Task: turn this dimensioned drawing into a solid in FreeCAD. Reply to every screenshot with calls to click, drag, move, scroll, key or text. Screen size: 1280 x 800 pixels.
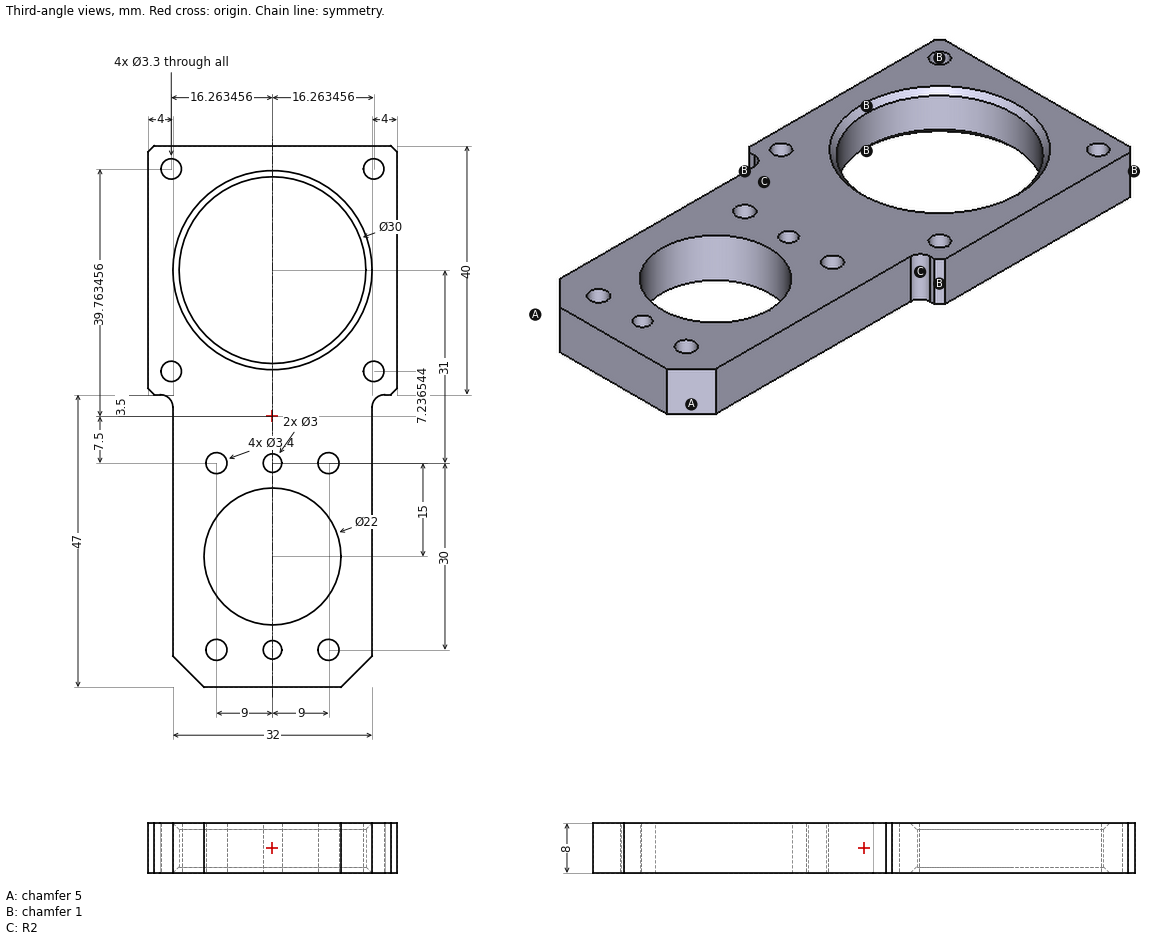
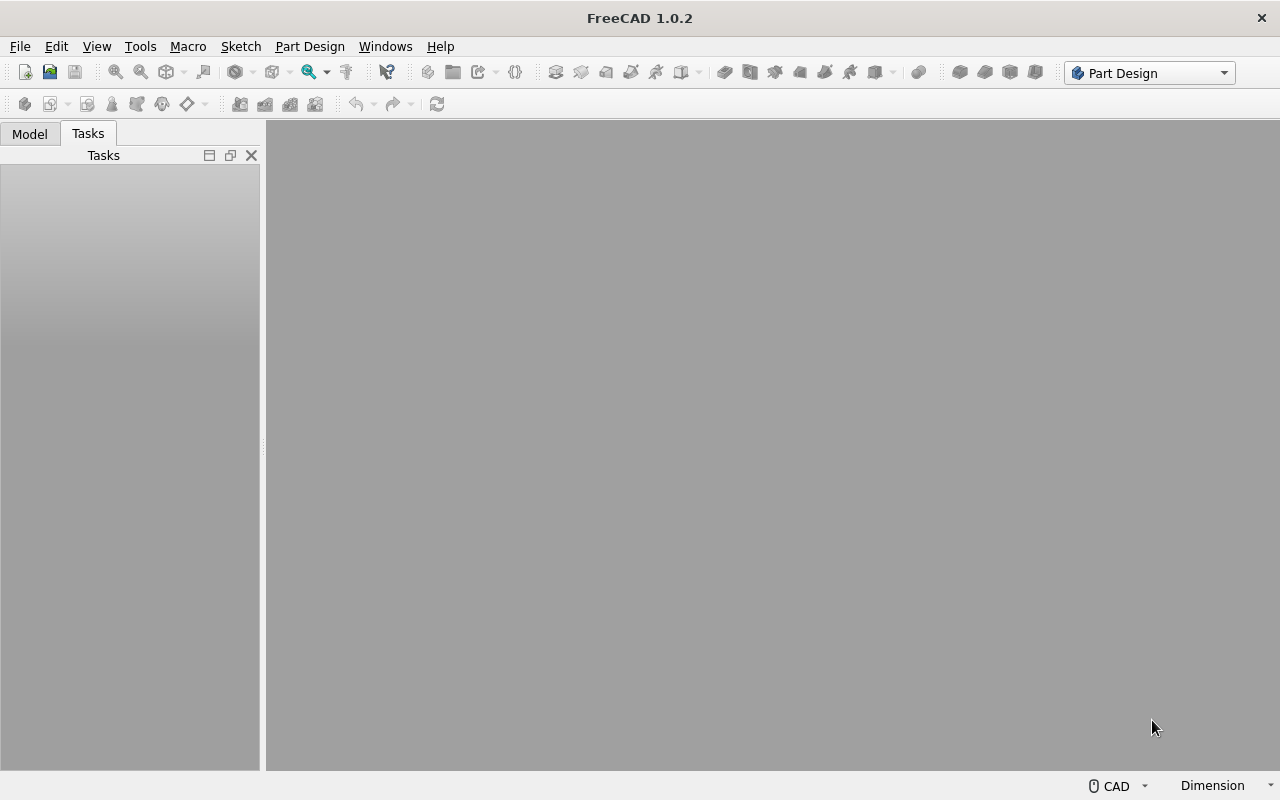
click(25, 72)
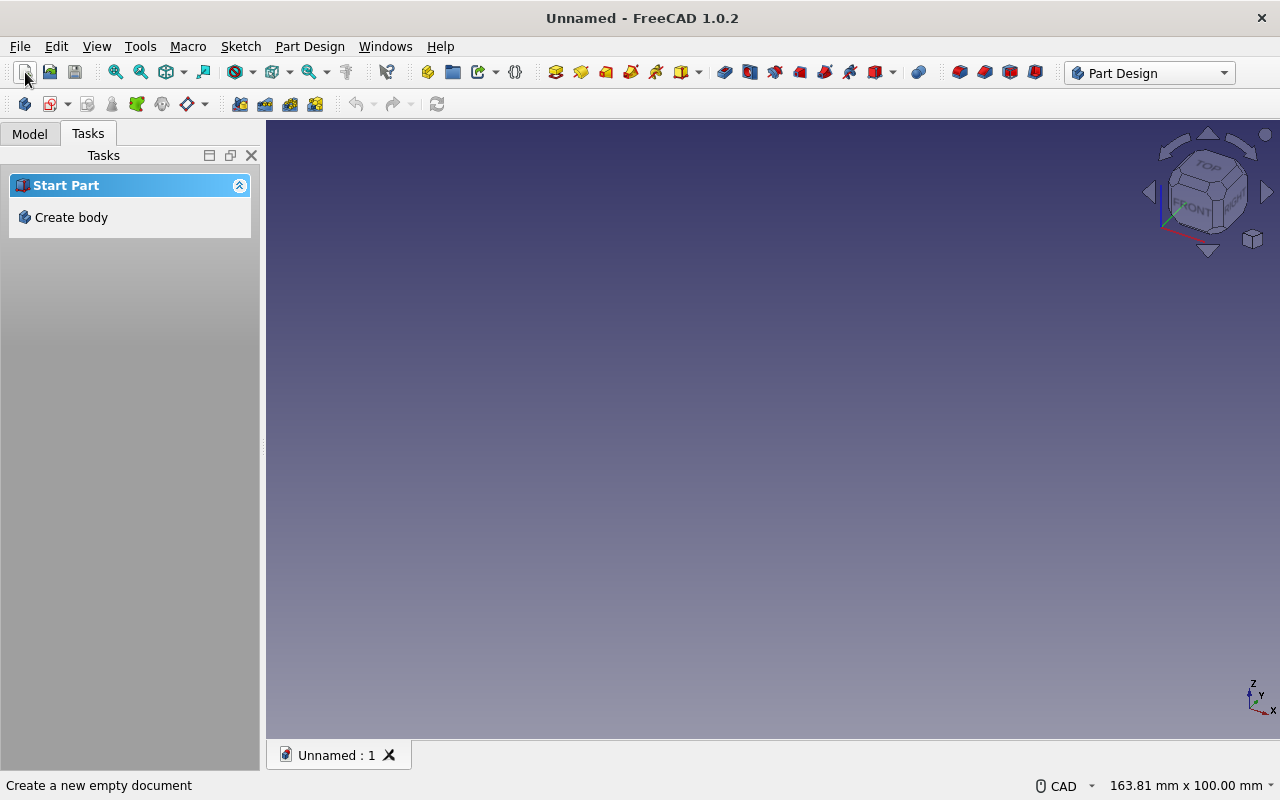
click(50, 104)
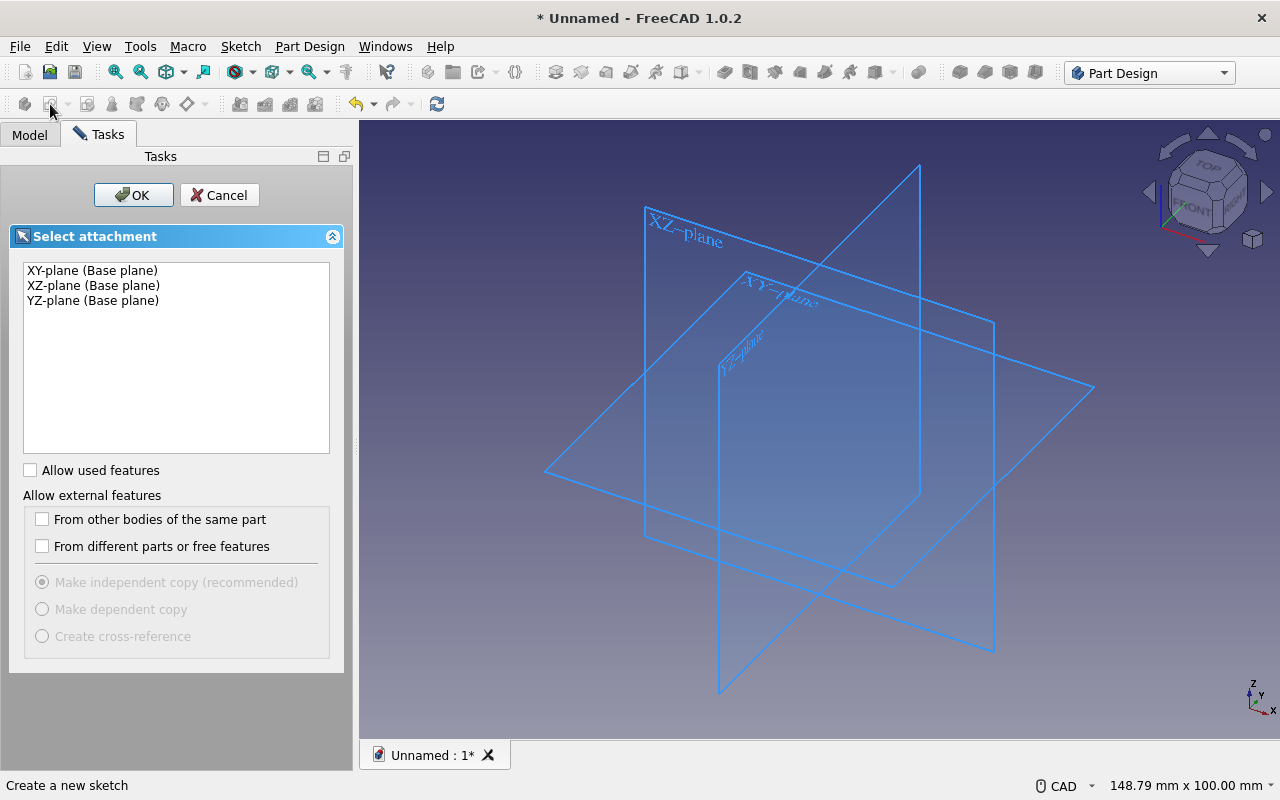
click(84, 270)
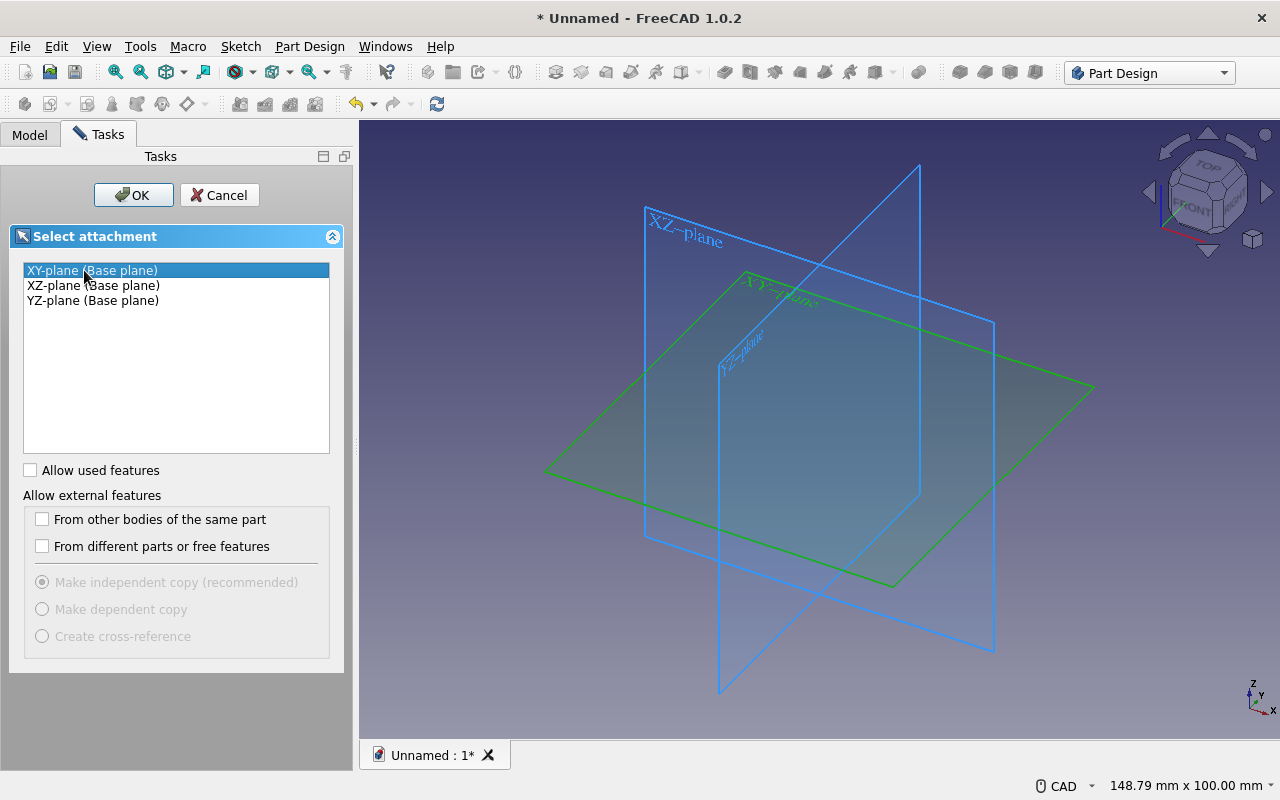
click(134, 195)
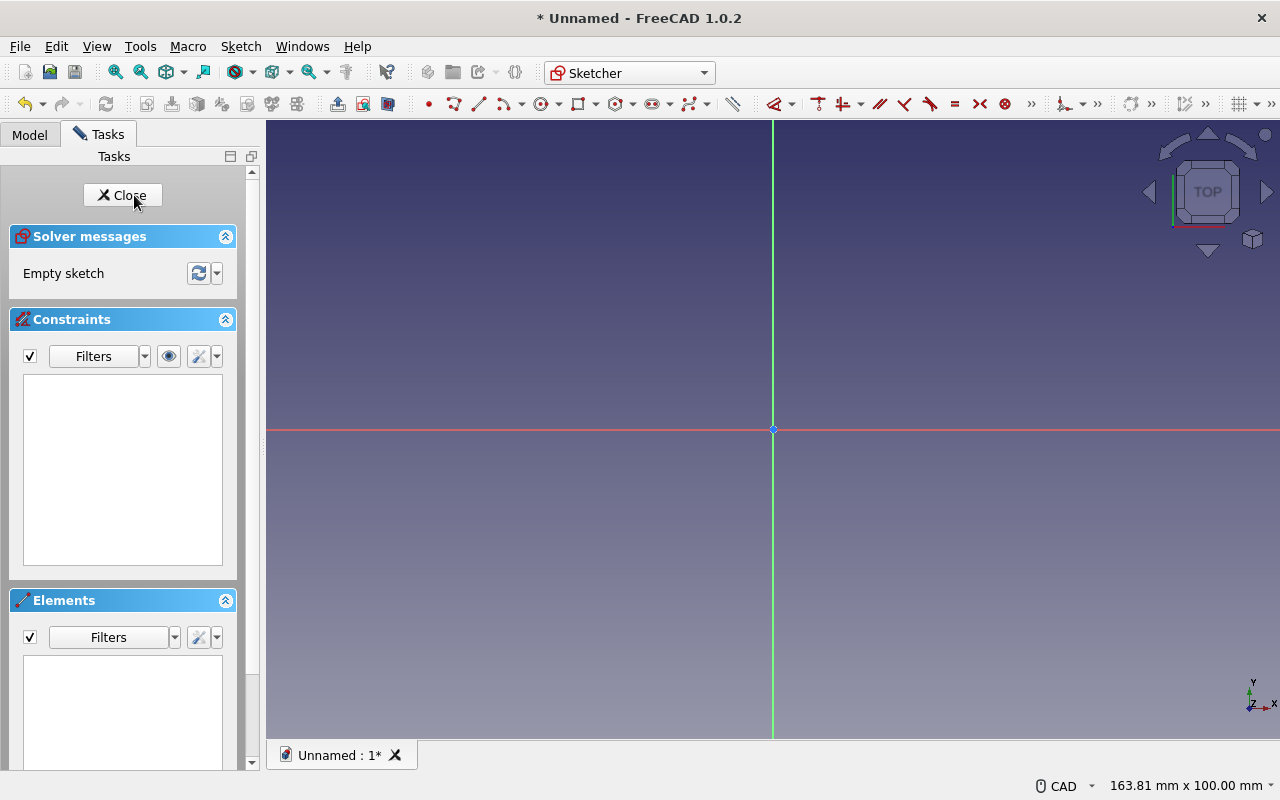
scroll(565, 429, down, 2)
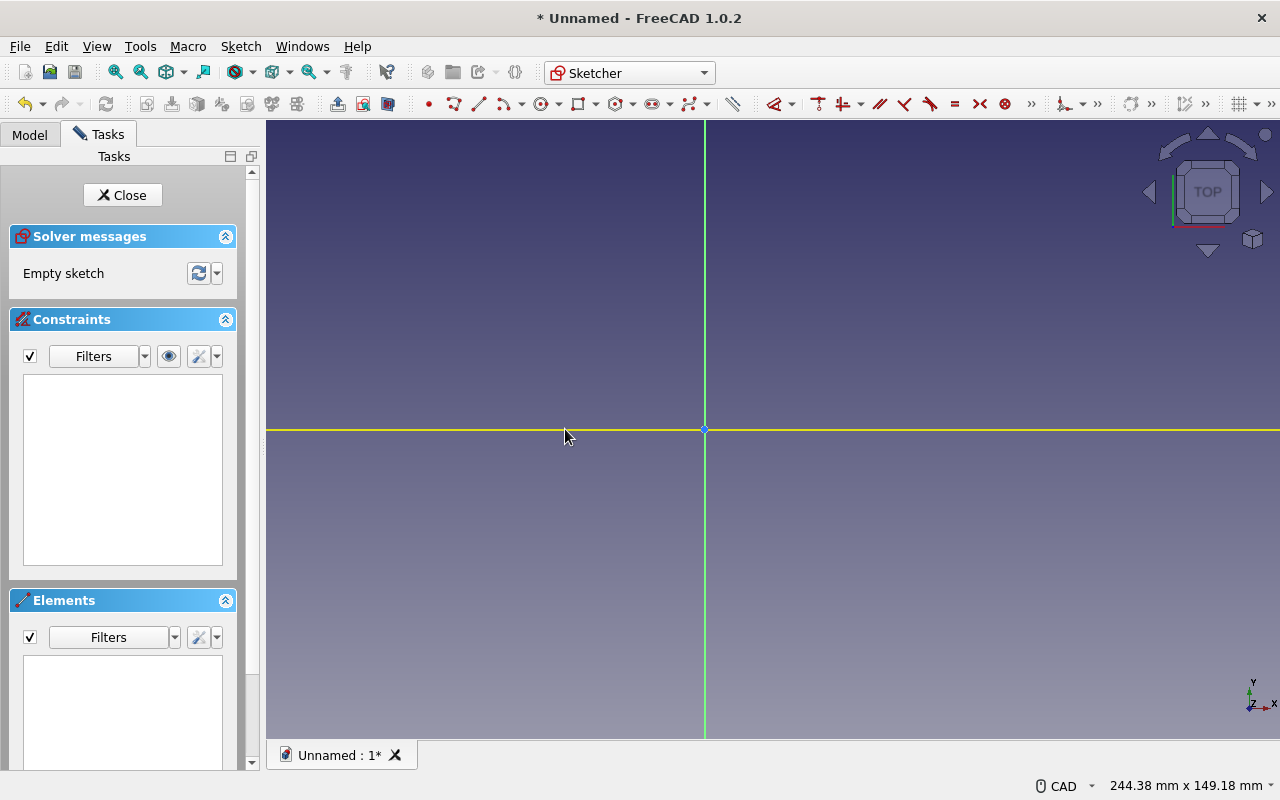
click(454, 104)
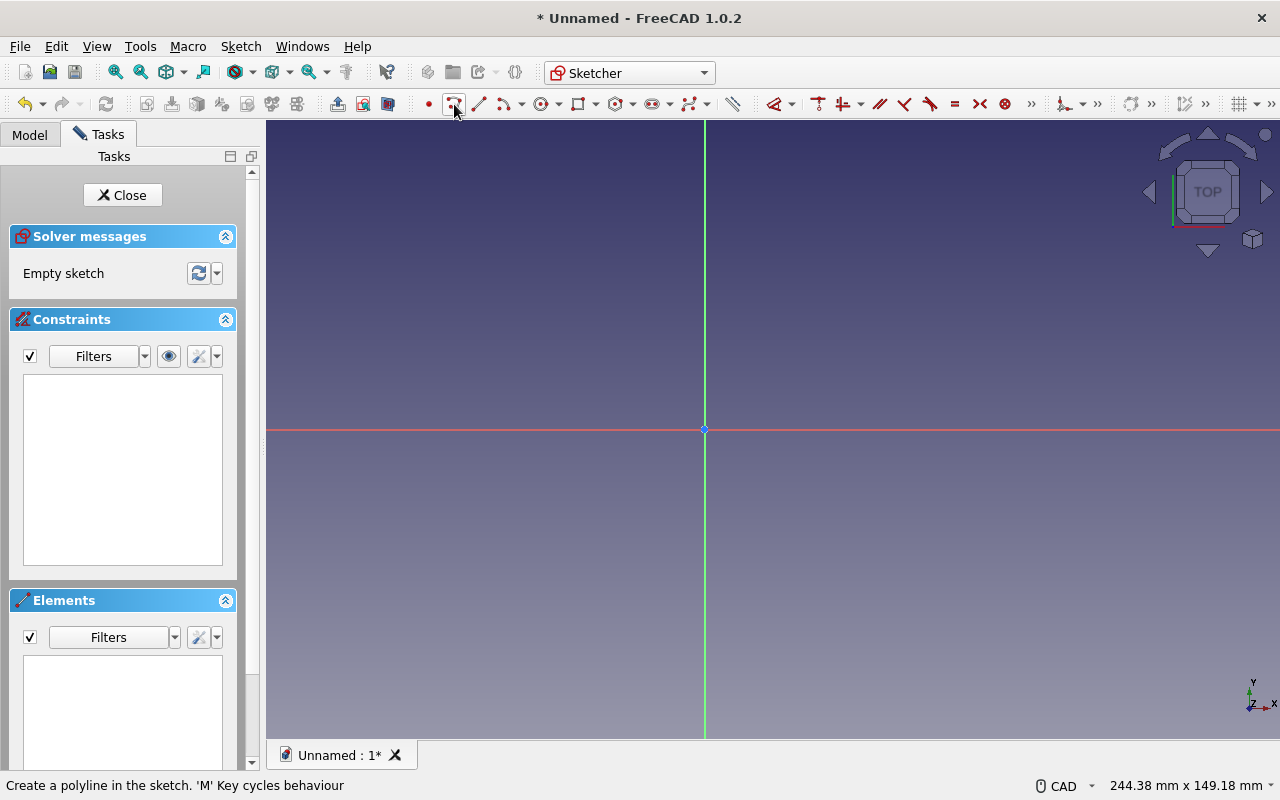
click(638, 415)
click(638, 610)
click(771, 610)
click(771, 415)
click(788, 415)
click(788, 249)
click(622, 249)
click(622, 415)
click(638, 416)
key(Escape)
key(Escape)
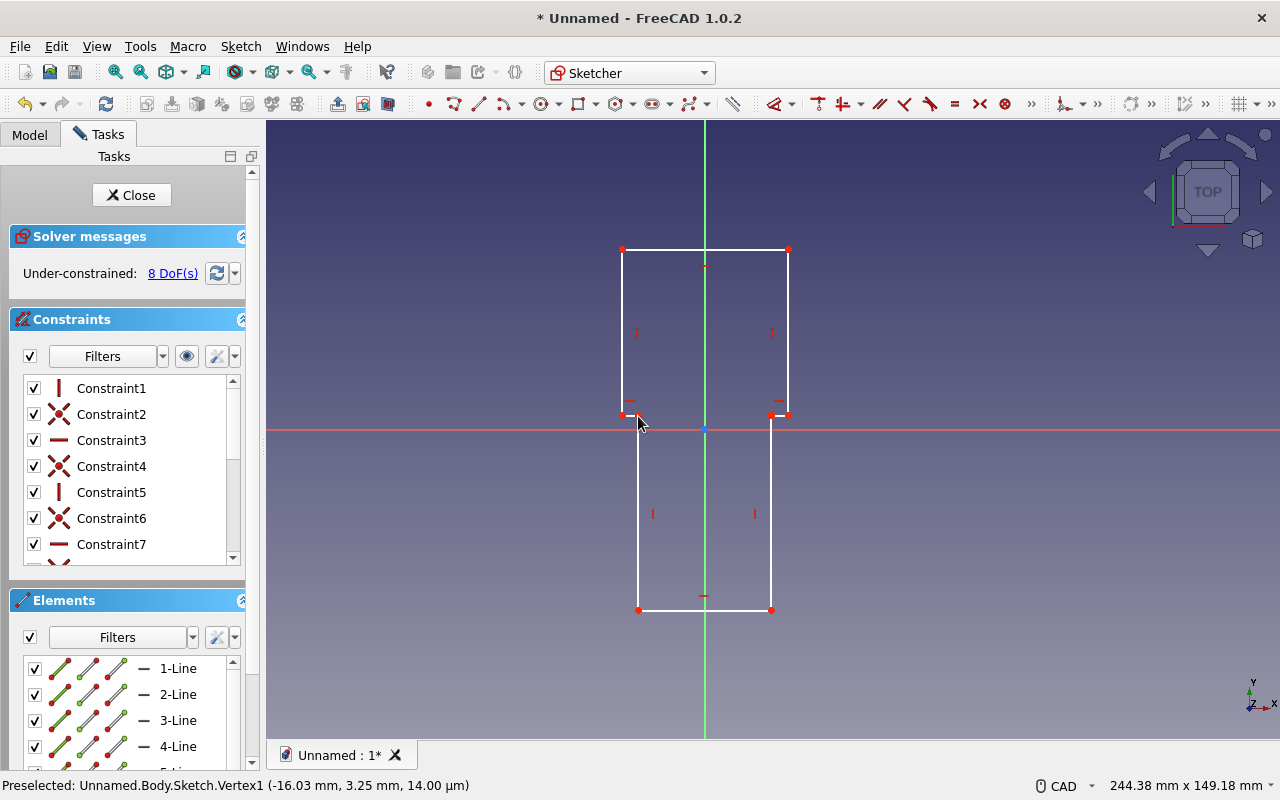
click(638, 416)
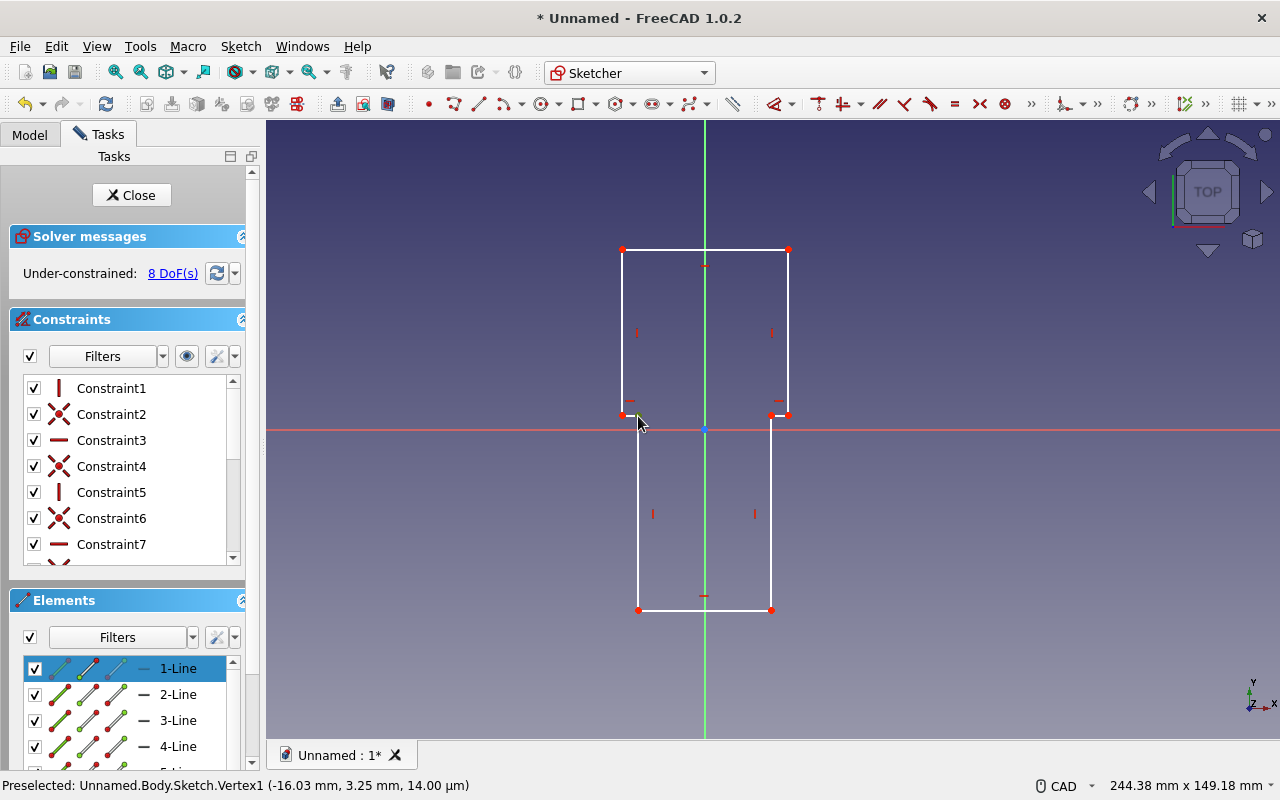
click(771, 416)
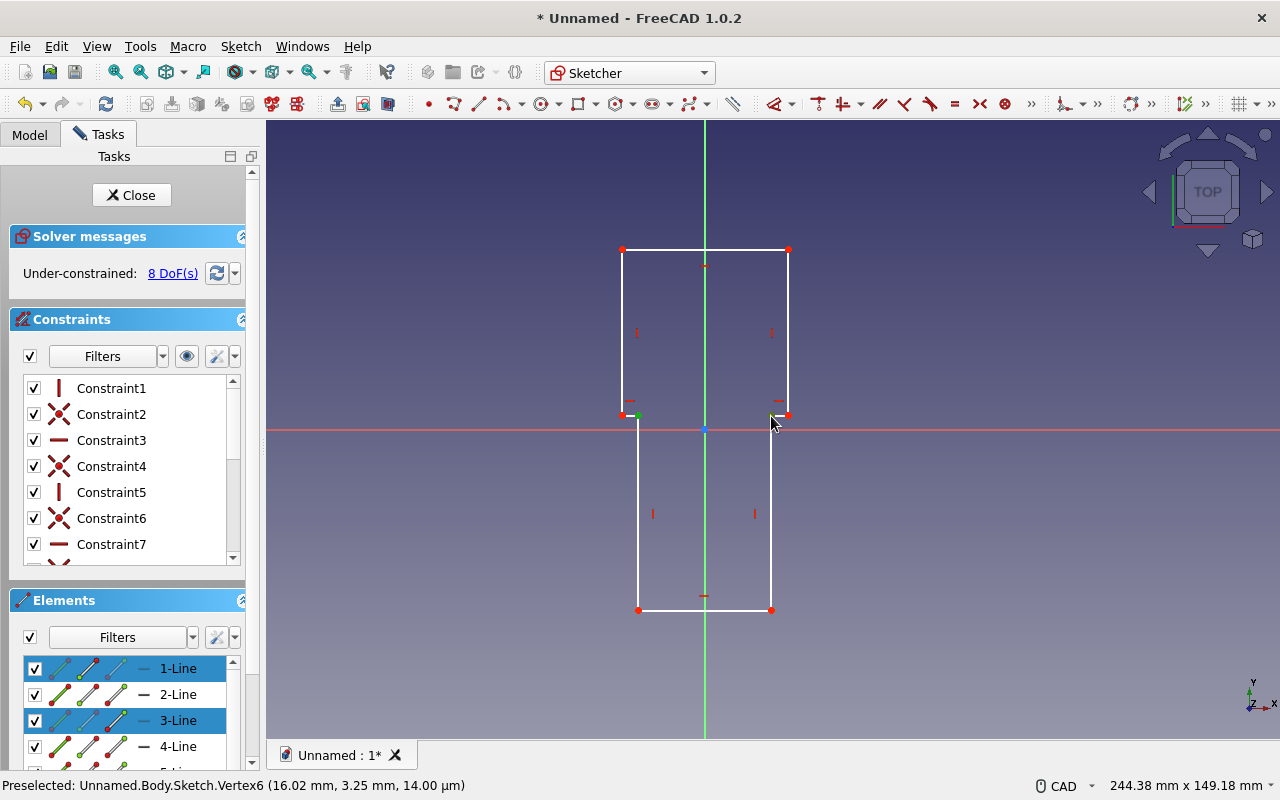
click(705, 671)